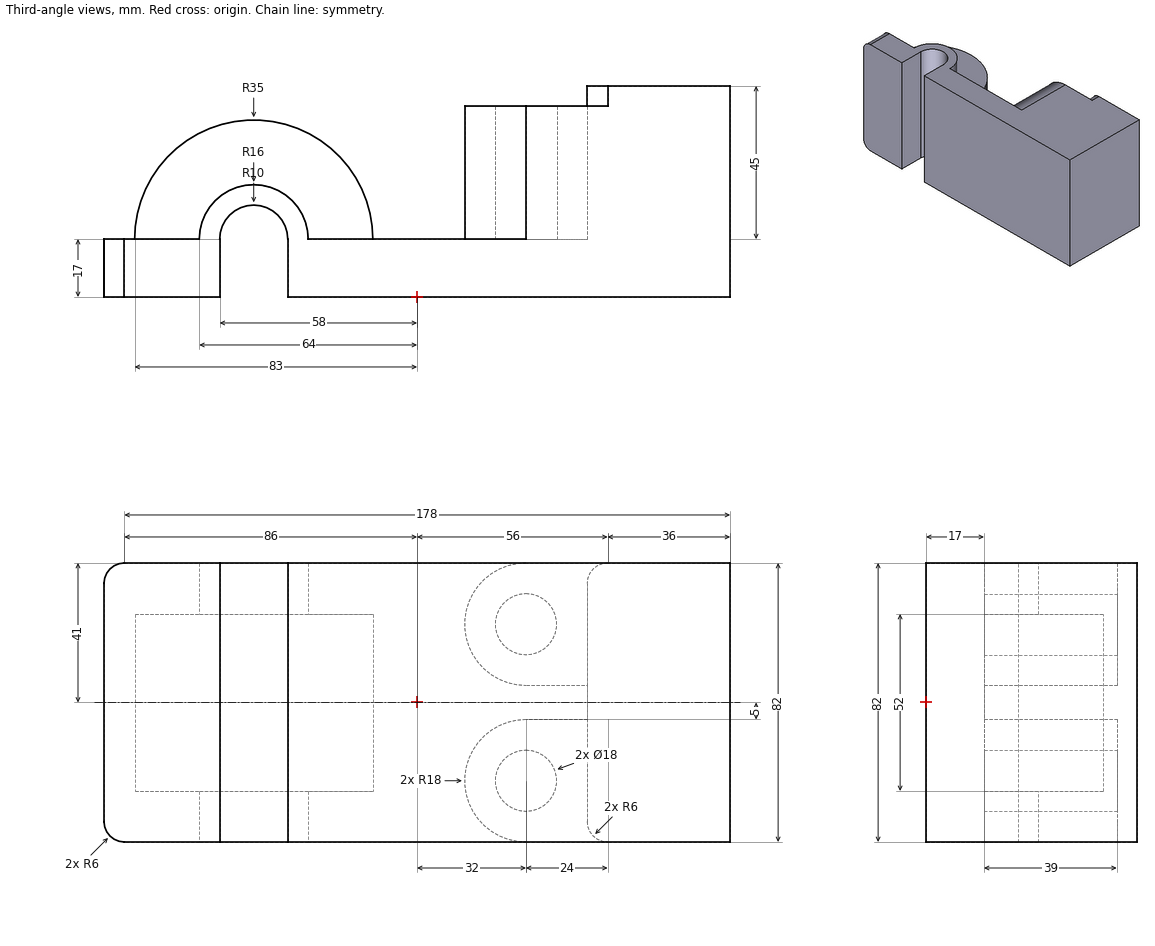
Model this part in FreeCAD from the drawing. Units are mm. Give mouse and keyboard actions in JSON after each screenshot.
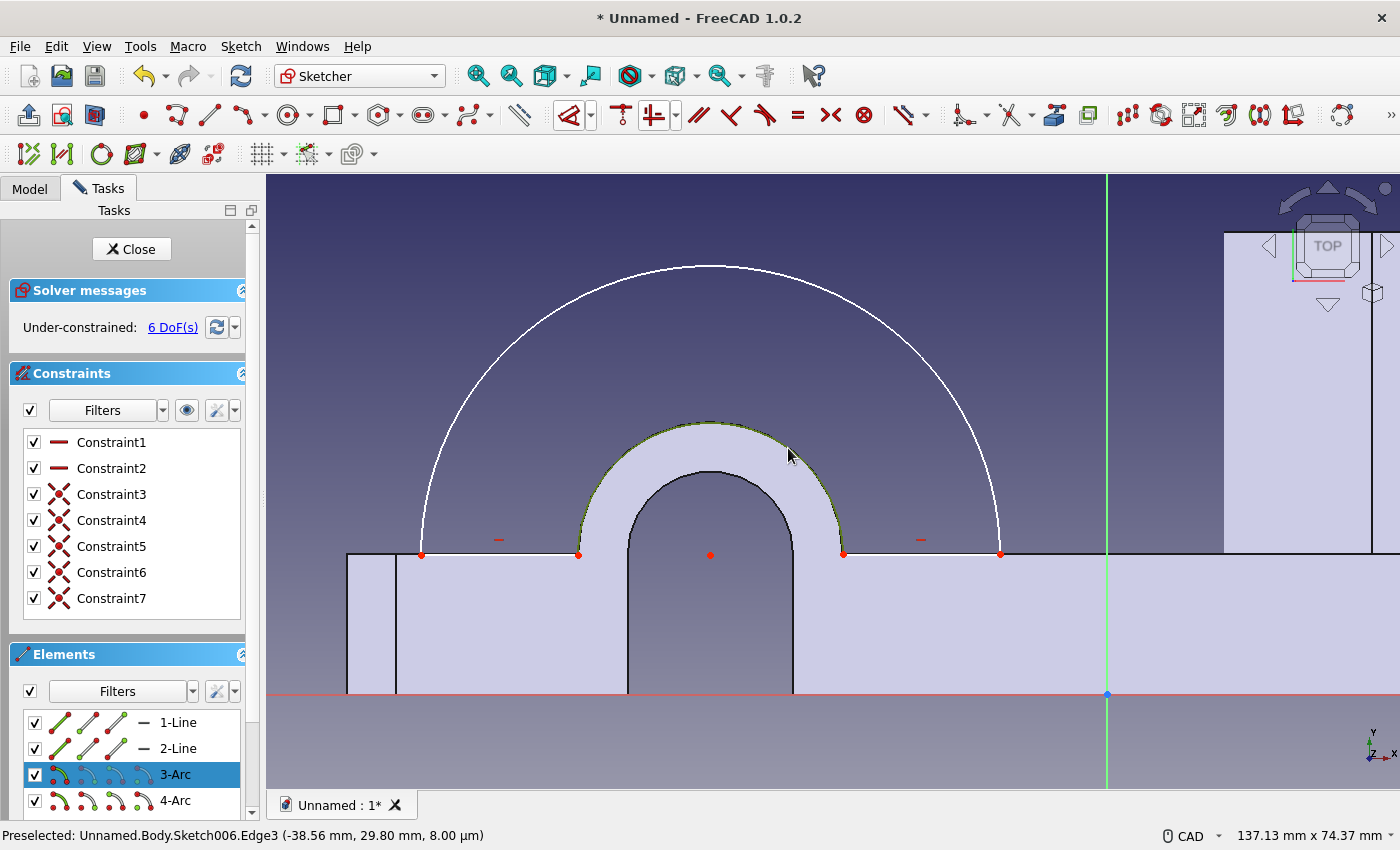
{"action": "key", "text": "k r"}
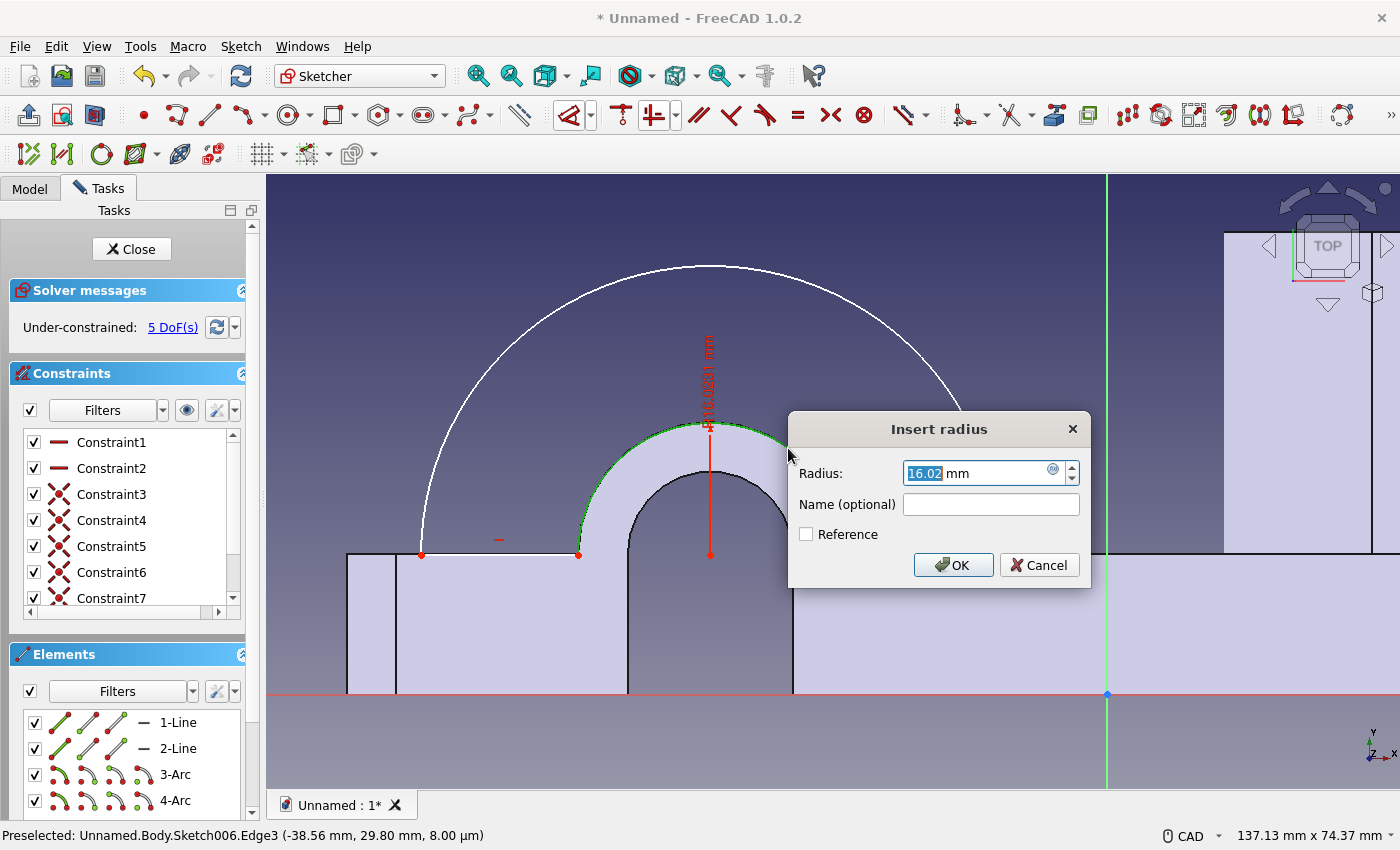
{"action": "type", "text": "16"}
{"action": "key", "text": "Return"}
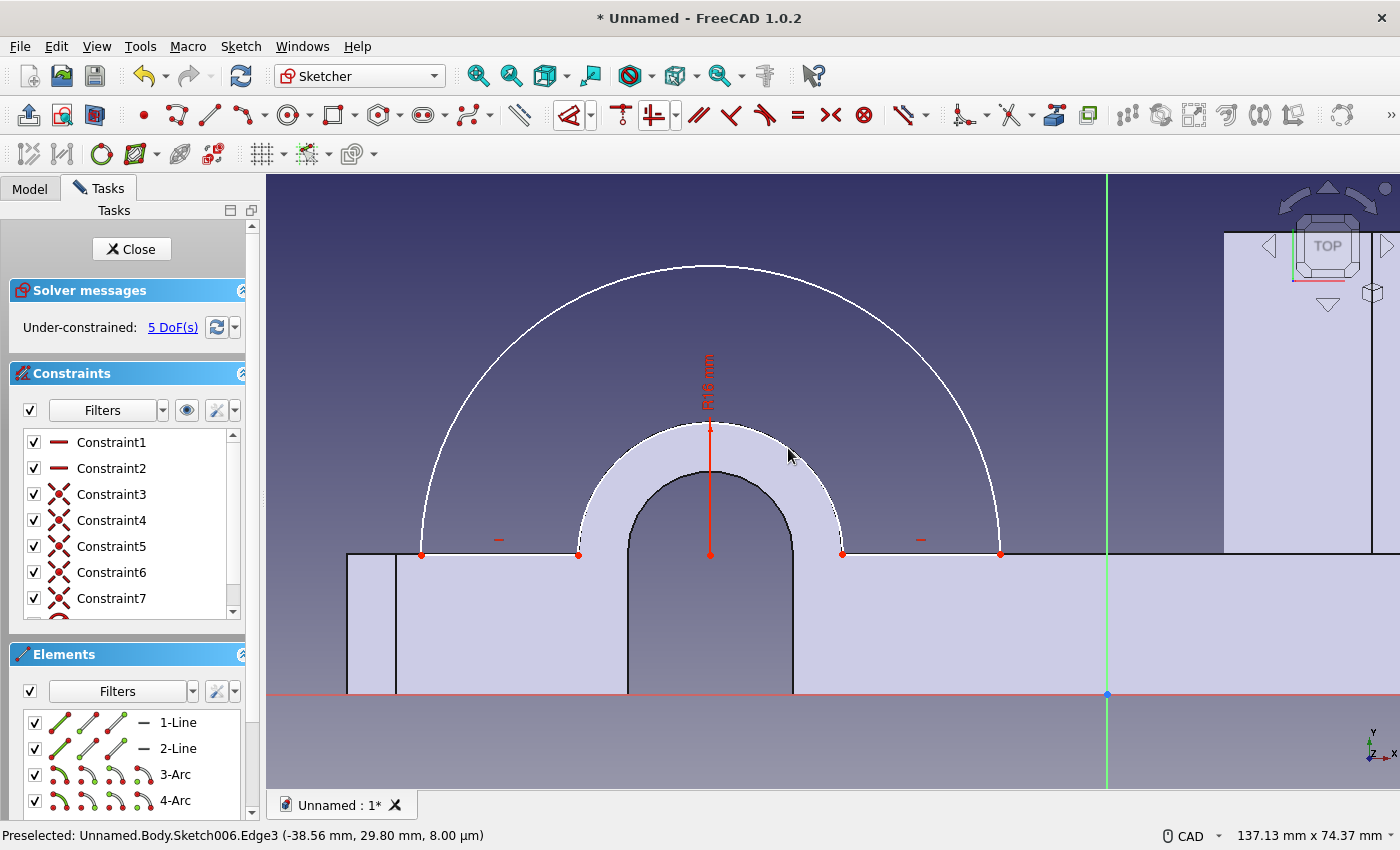
{"action": "left_click", "coordinate": [881, 321]}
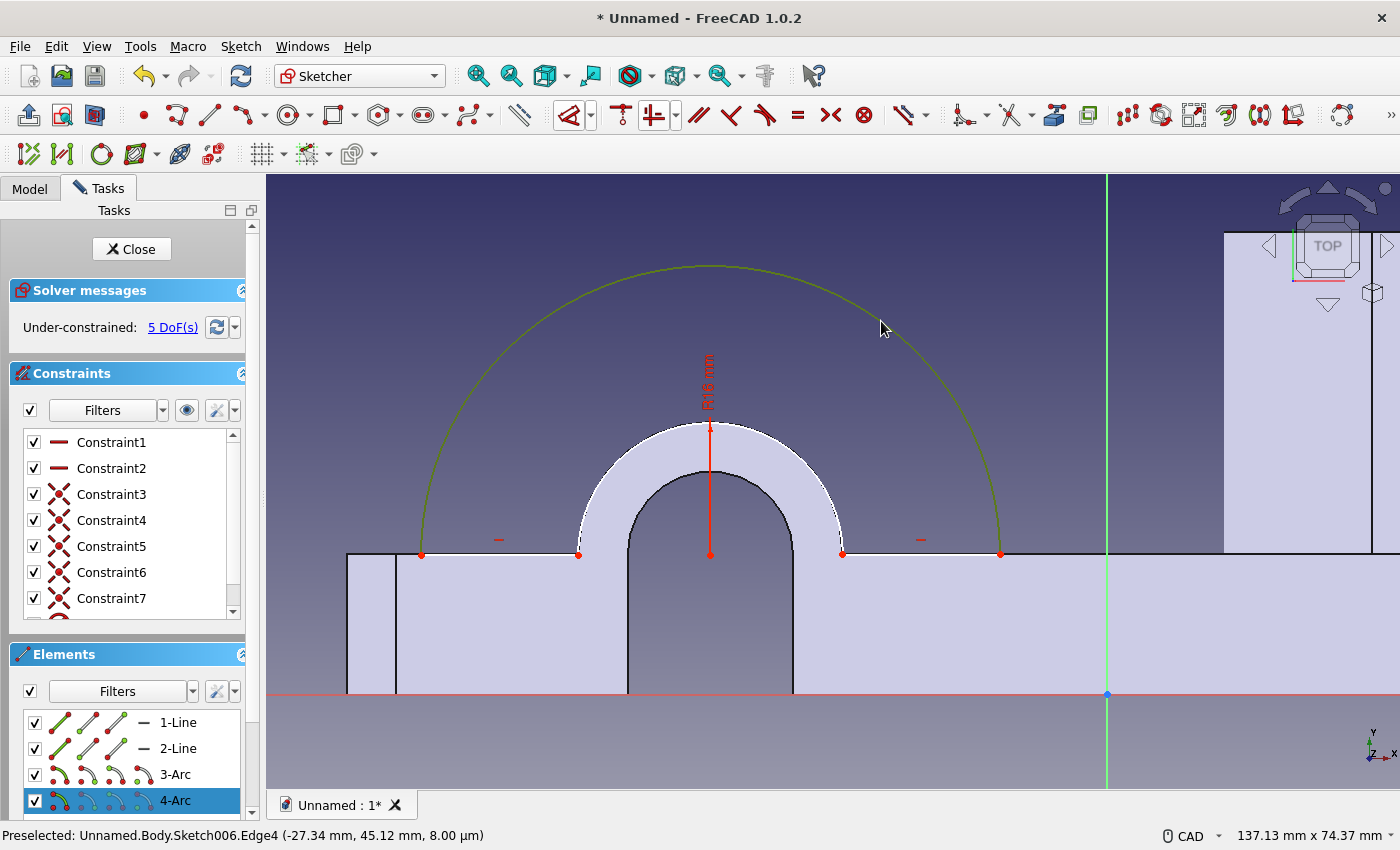
{"action": "left_click", "coordinate": [590, 116]}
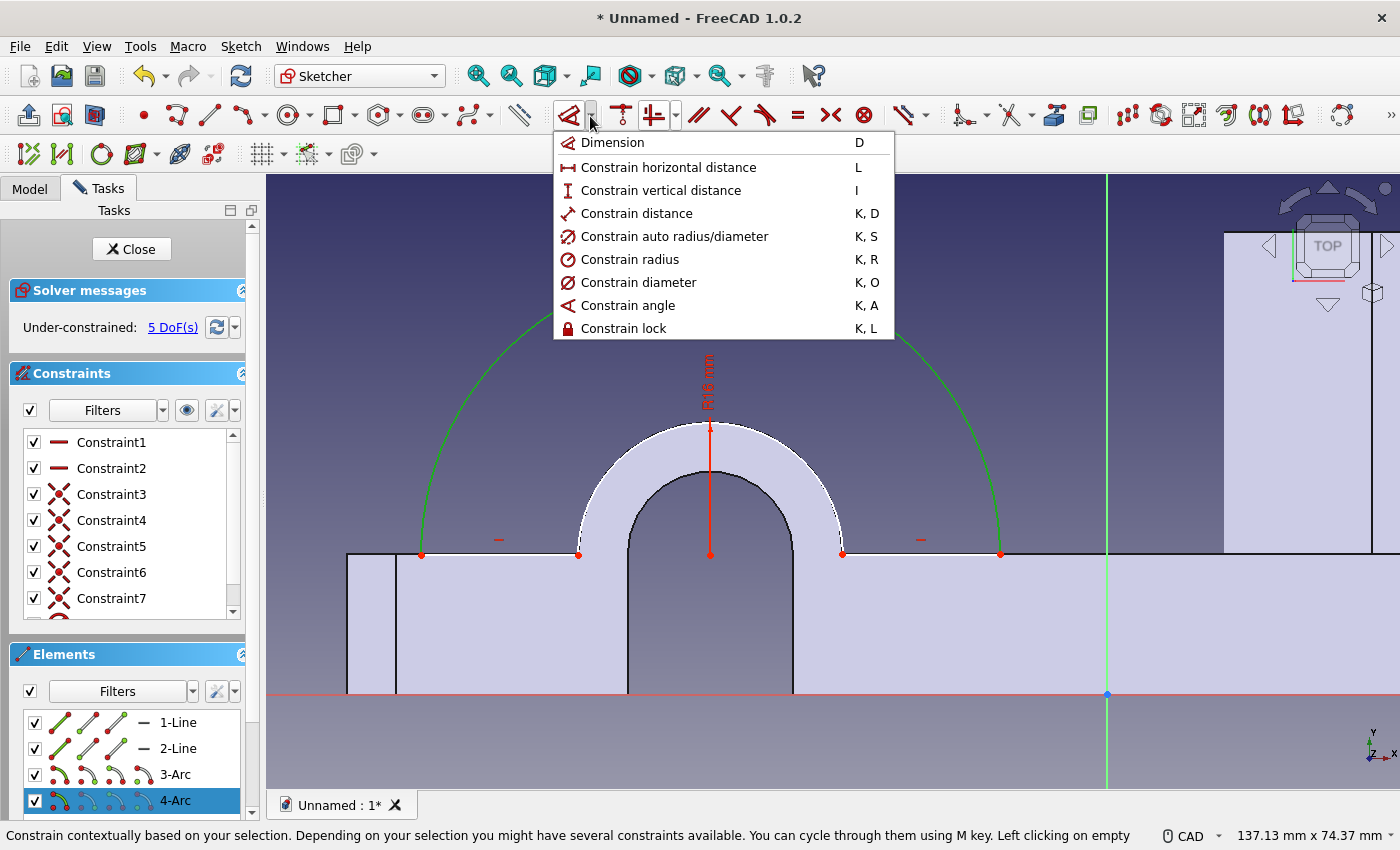
{"action": "left_click", "coordinate": [724, 260]}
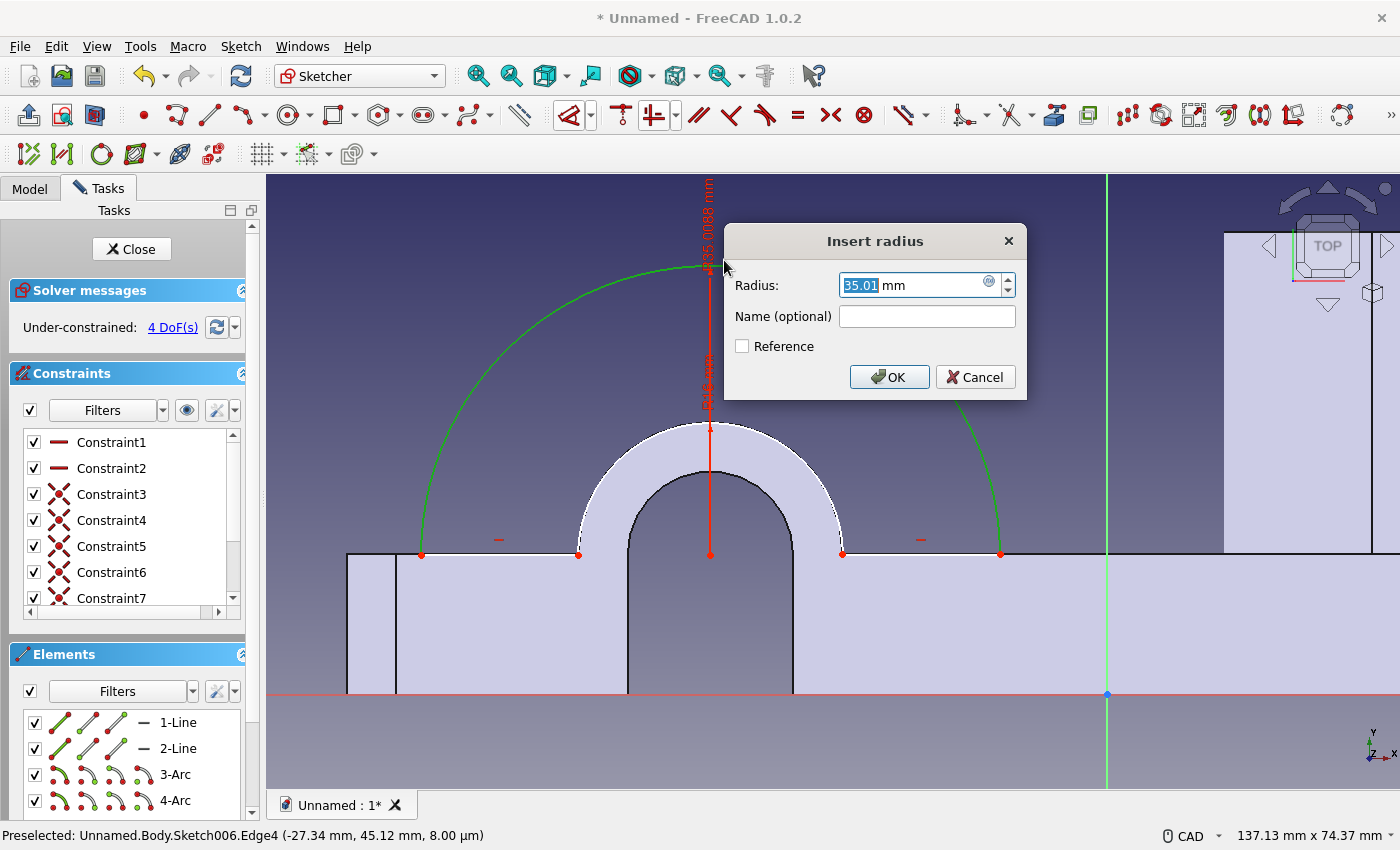
{"action": "type", "text": "35"}
{"action": "key", "text": "Return"}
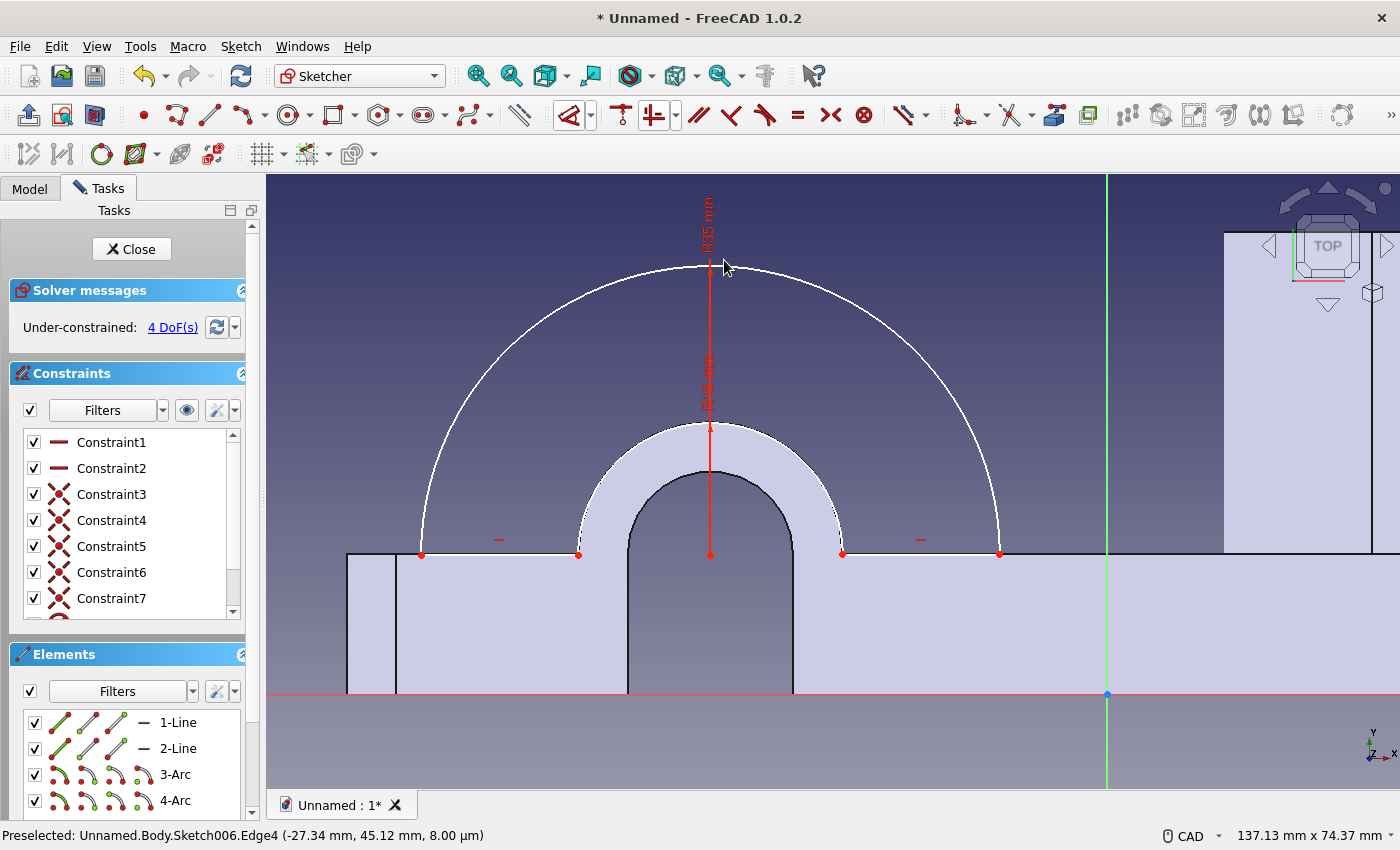
{"action": "left_click", "coordinate": [421, 555]}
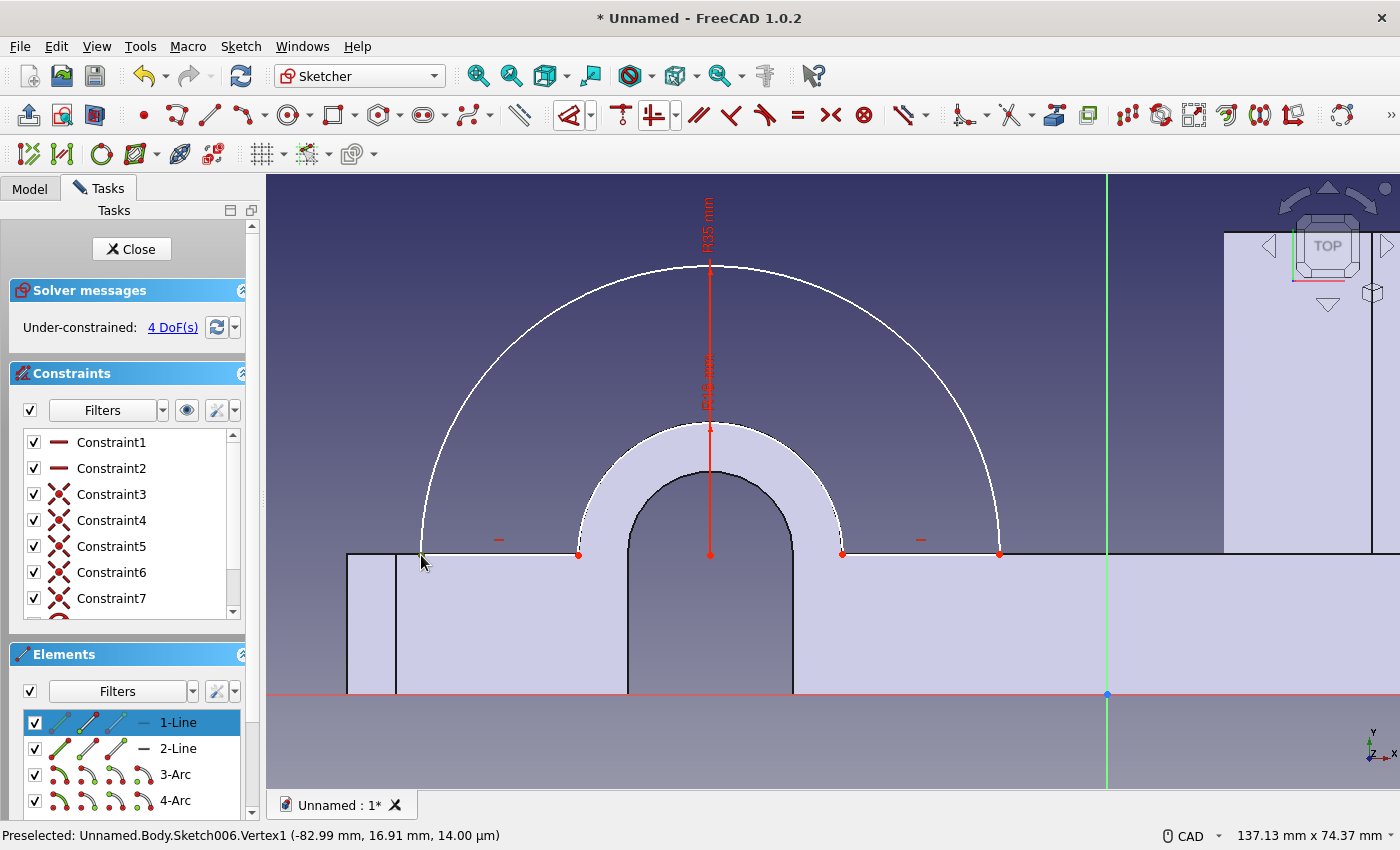
{"action": "key", "text": "l"}